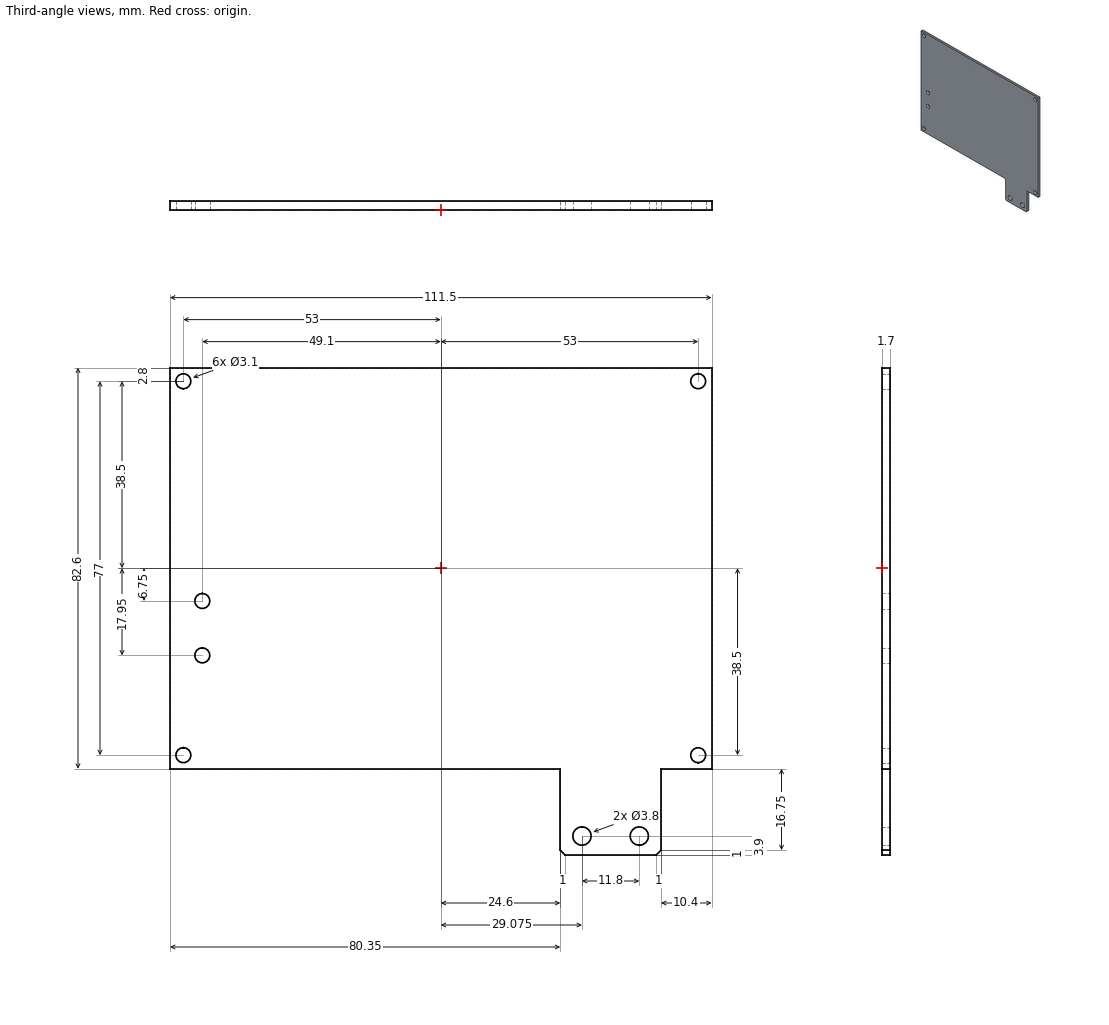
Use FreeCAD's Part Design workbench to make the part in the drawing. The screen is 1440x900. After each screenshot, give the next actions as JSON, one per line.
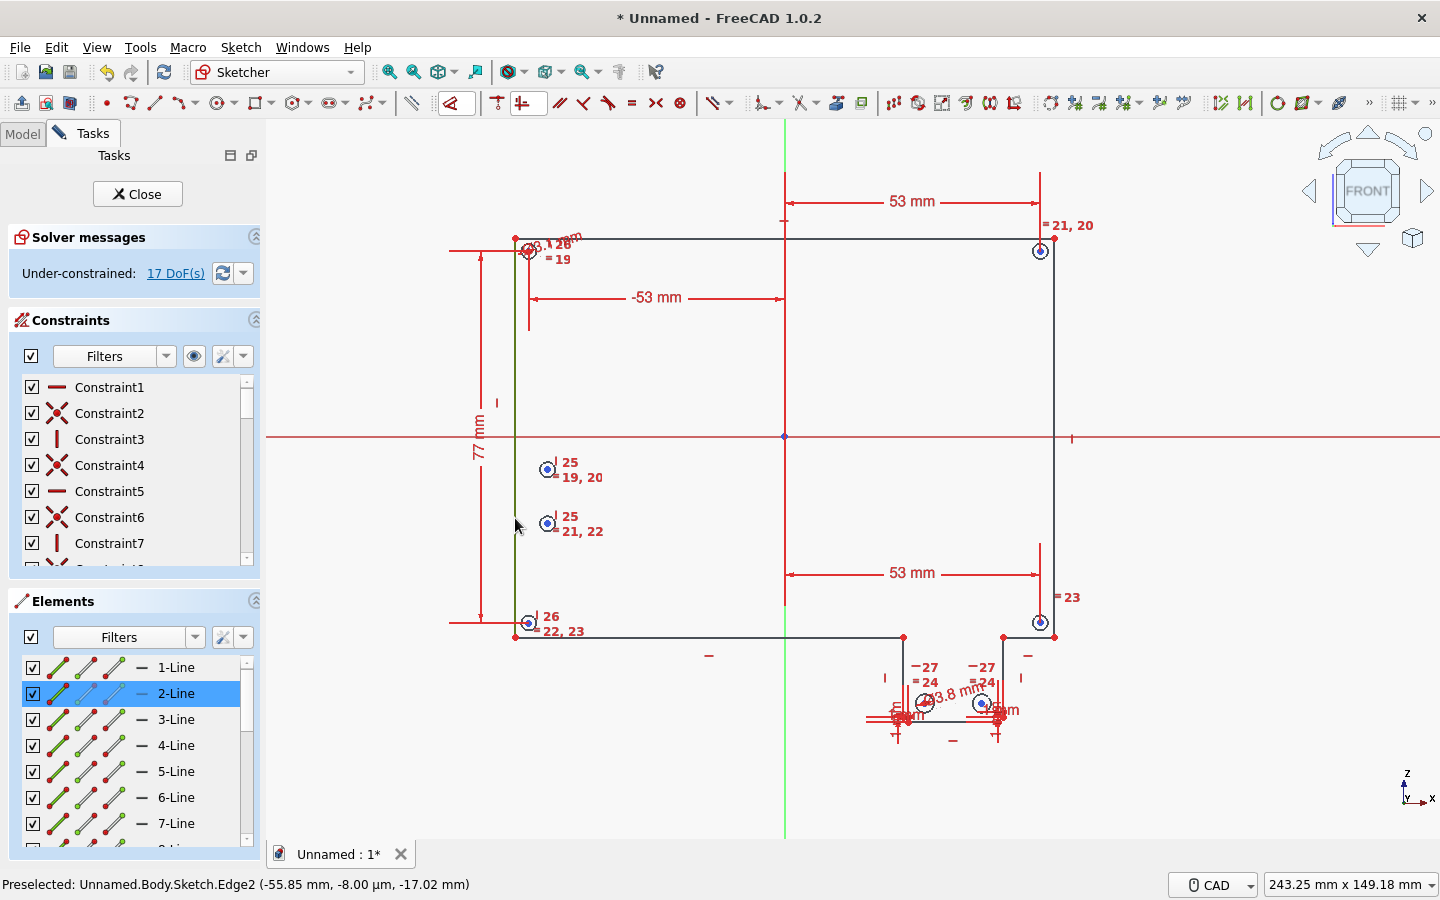
{"action": "key", "text": "i"}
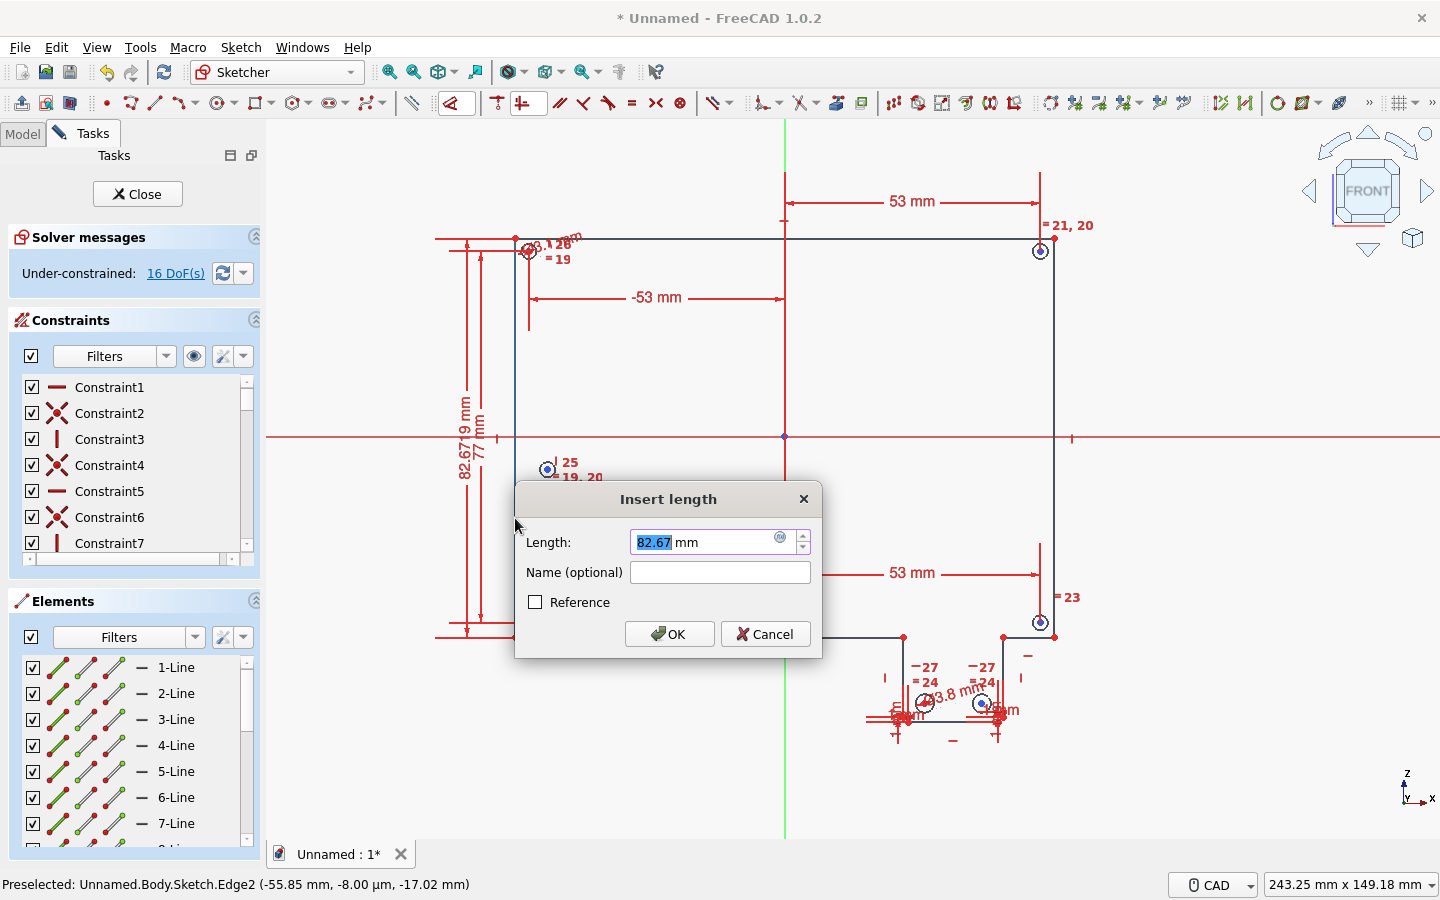
{"action": "type", "text": "82.6"}
{"action": "key", "text": "Return"}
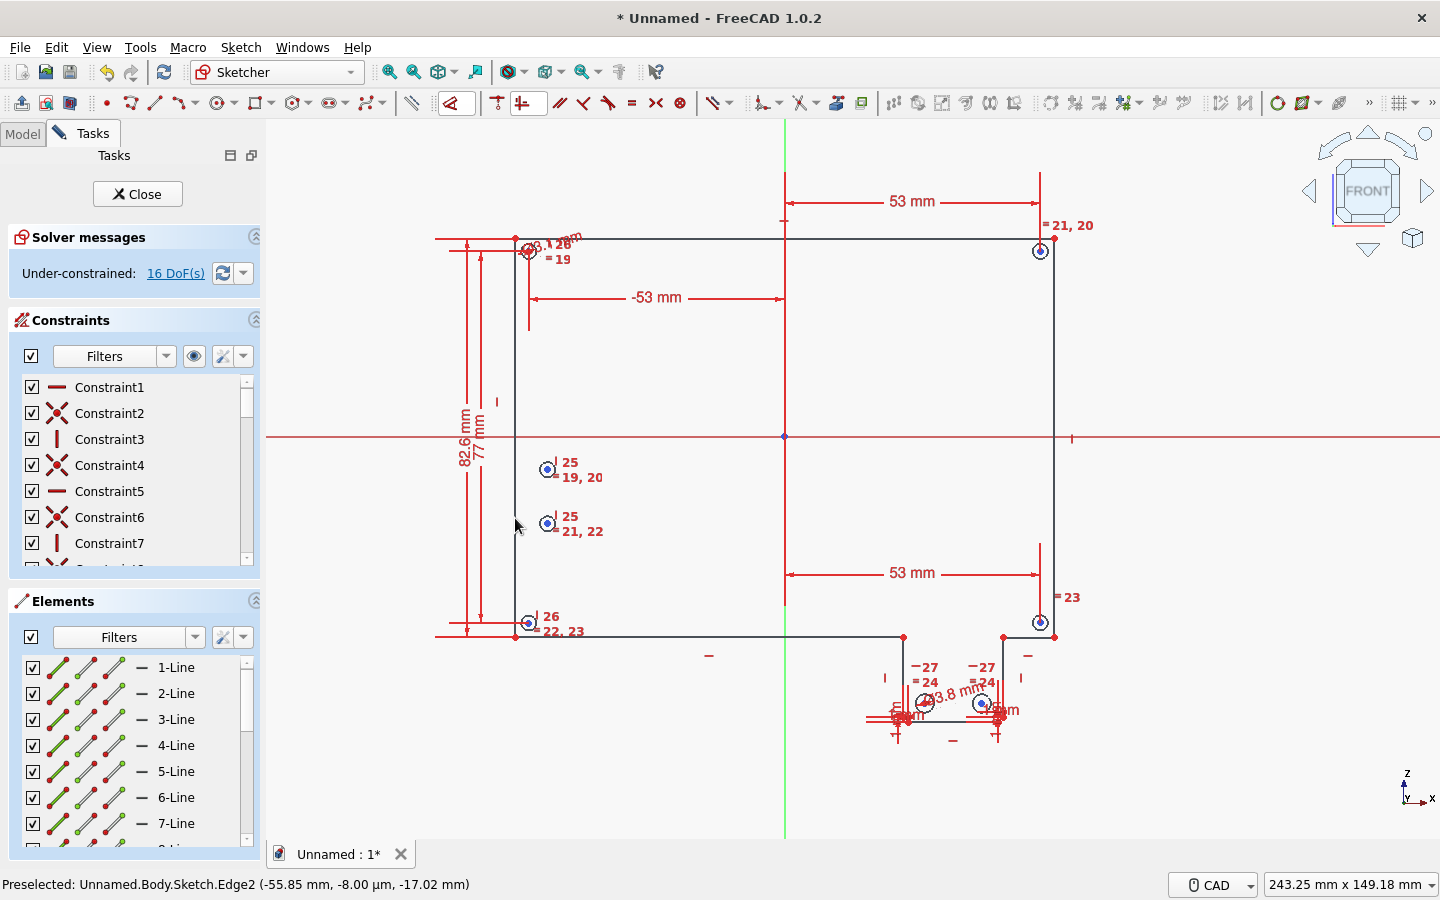
{"action": "left_click", "coordinate": [1054, 358]}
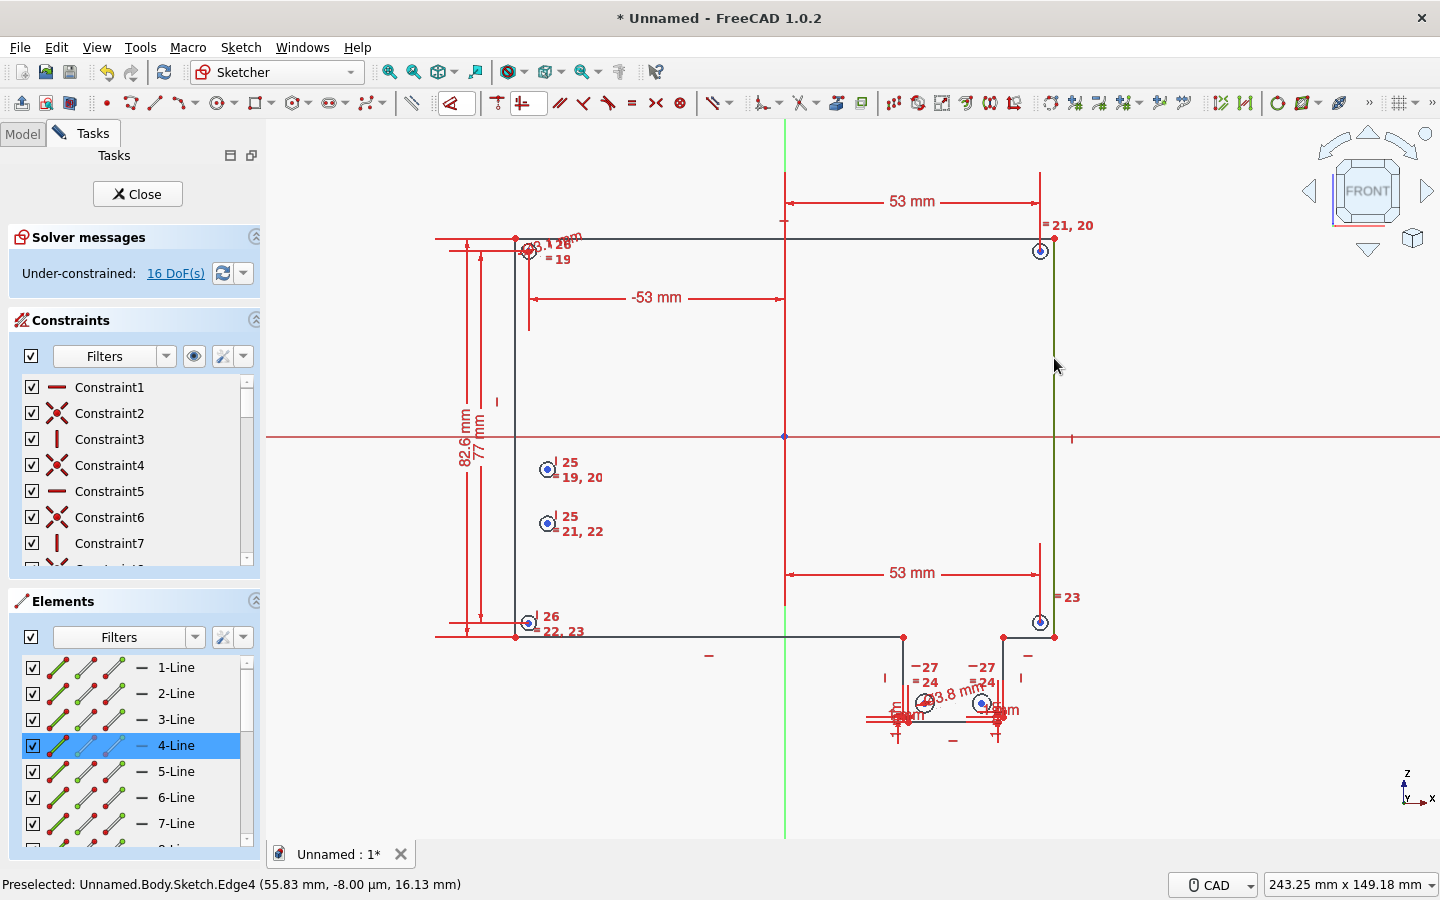
{"action": "key", "text": "i"}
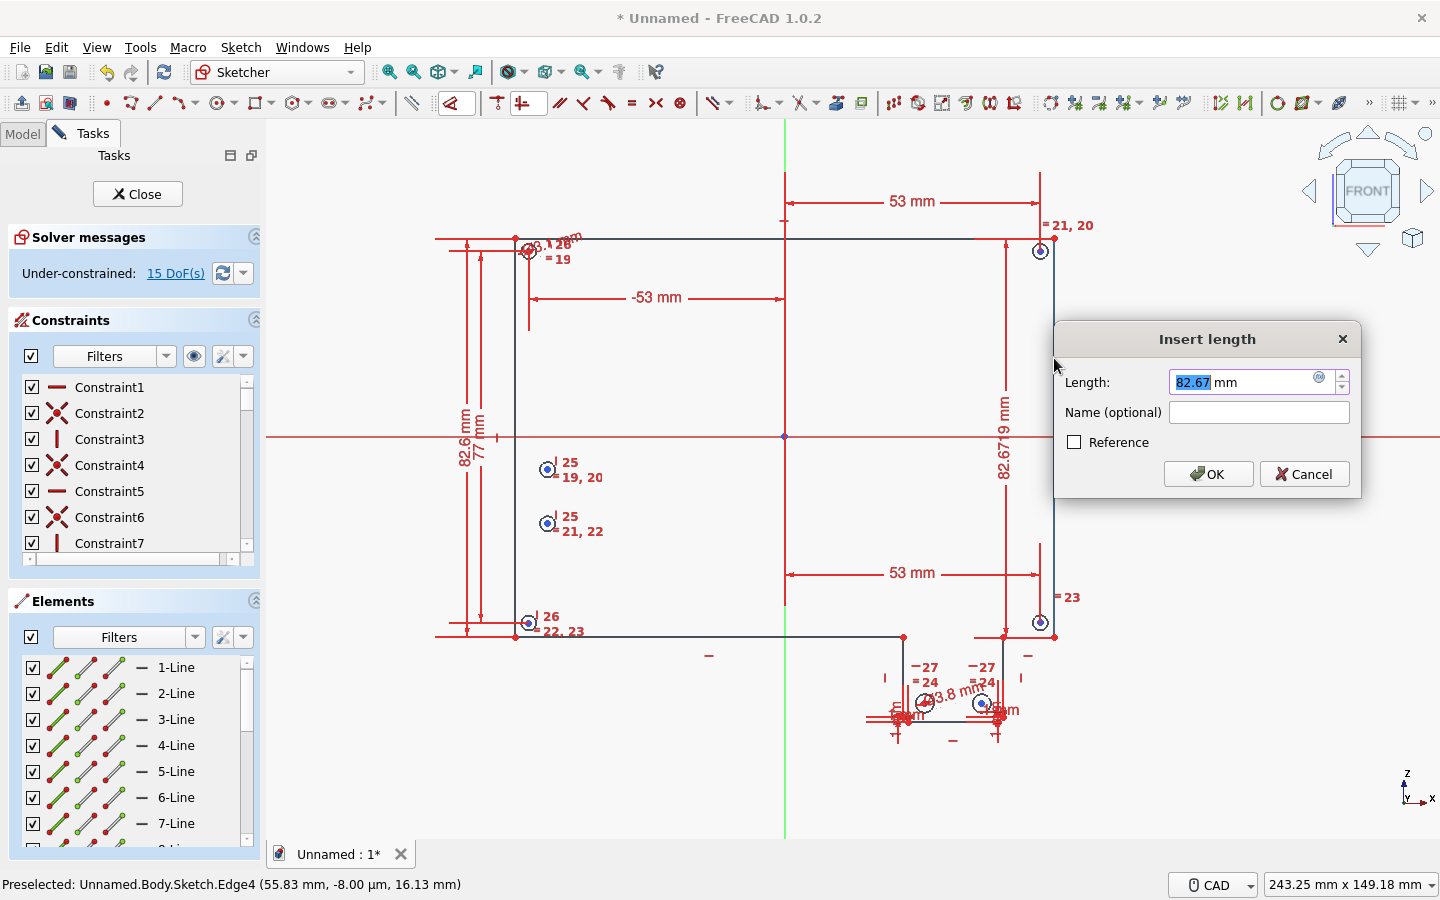
{"action": "type", "text": "82.6"}
{"action": "key", "text": "Return"}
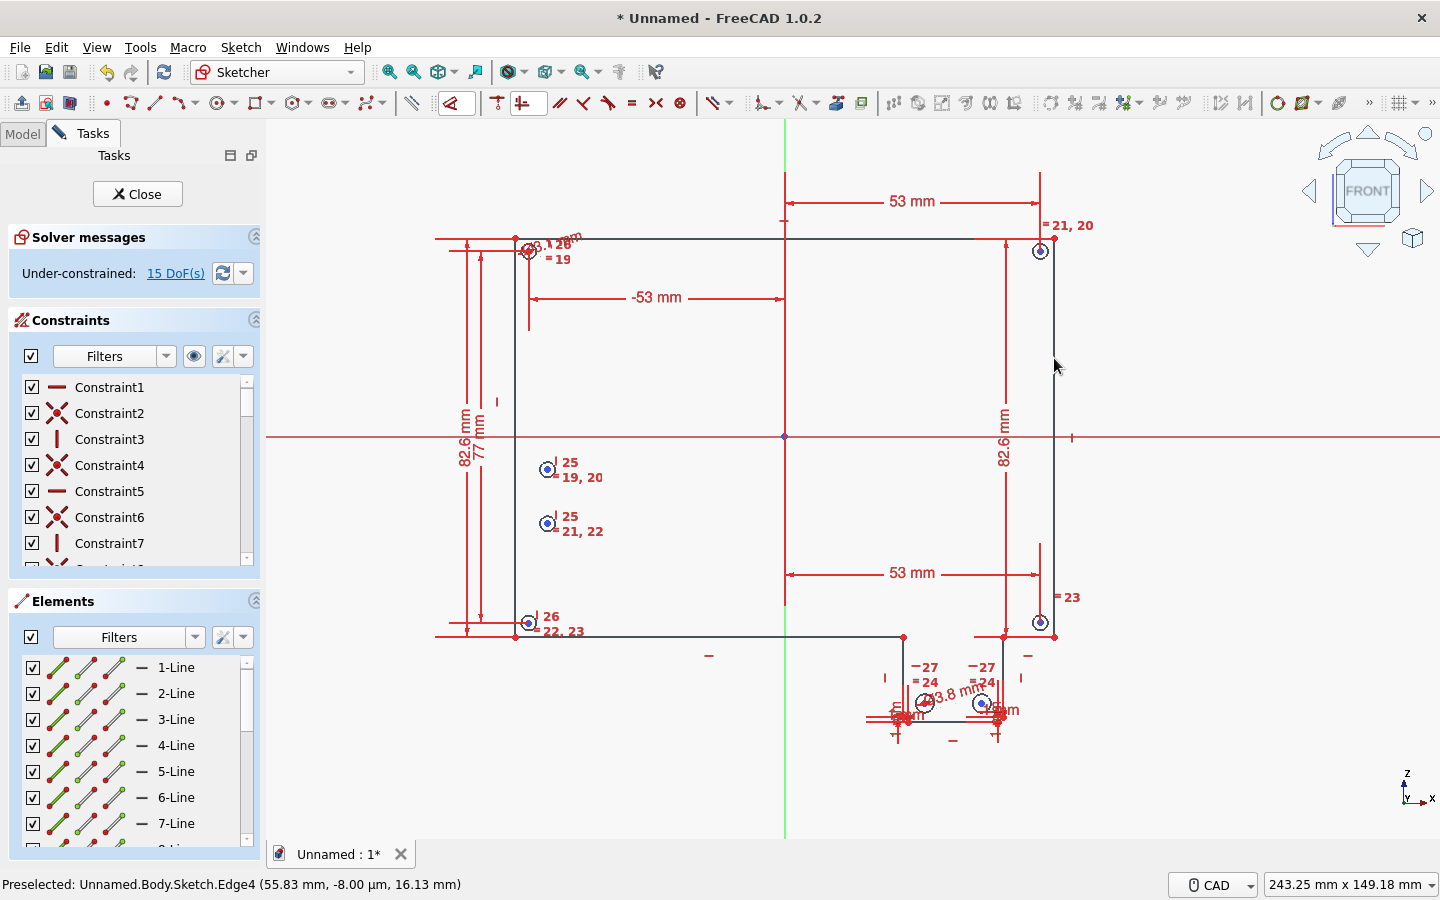
{"action": "left_click", "coordinate": [1018, 637]}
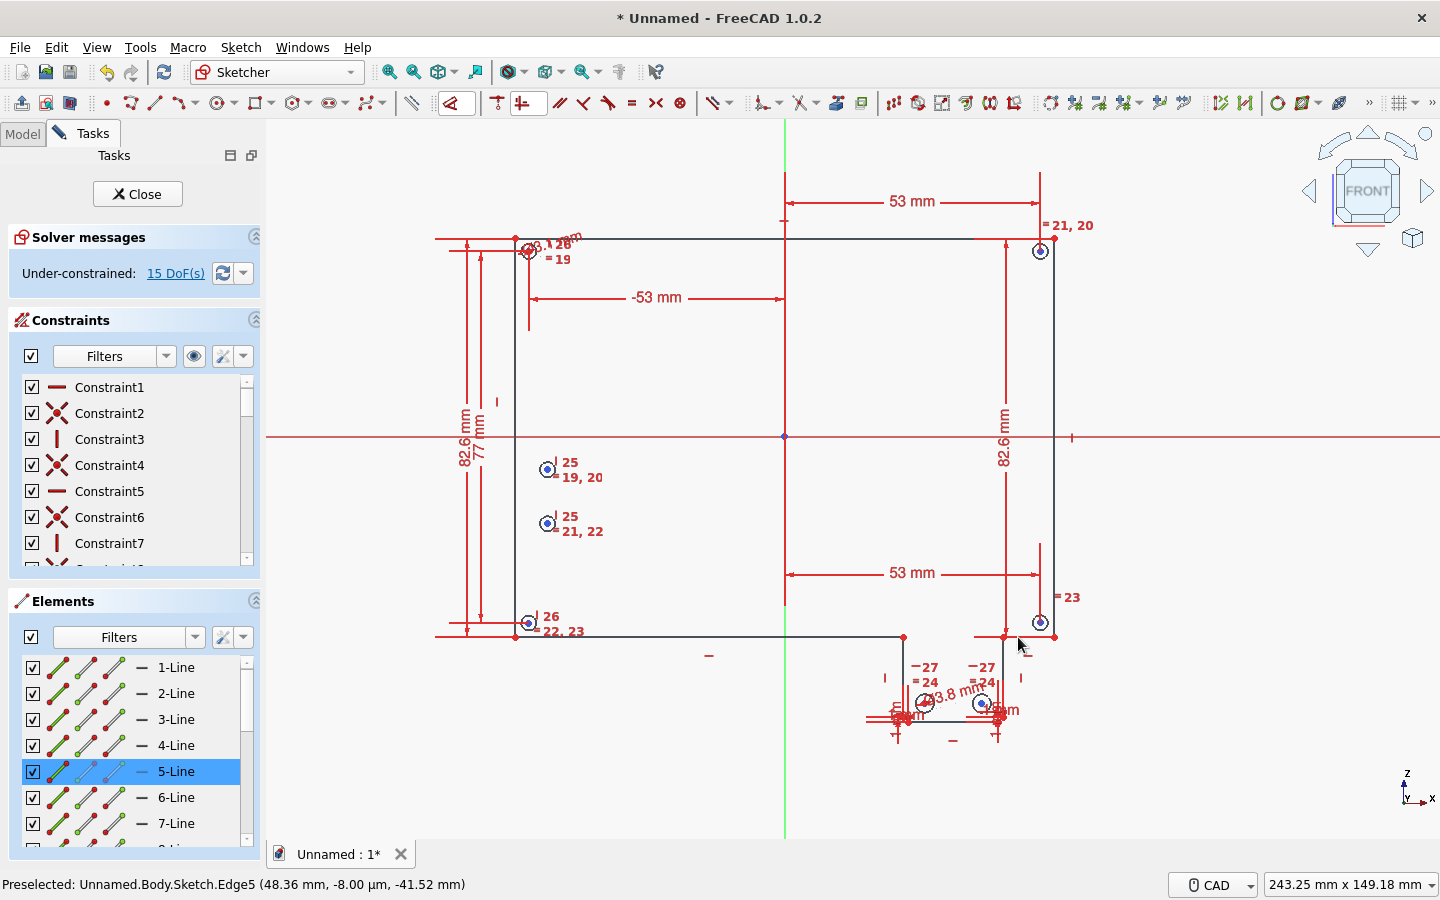
{"action": "key", "text": "l"}